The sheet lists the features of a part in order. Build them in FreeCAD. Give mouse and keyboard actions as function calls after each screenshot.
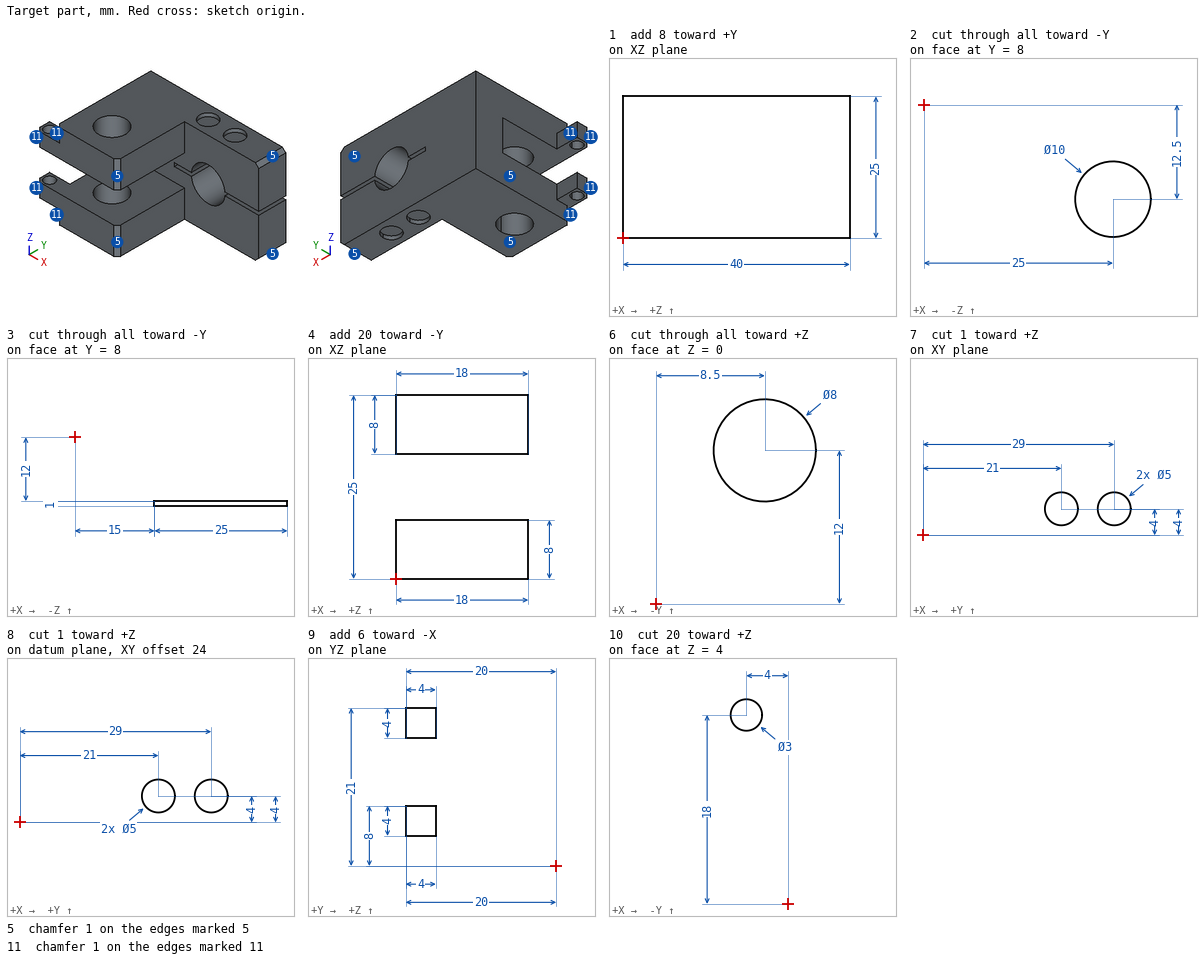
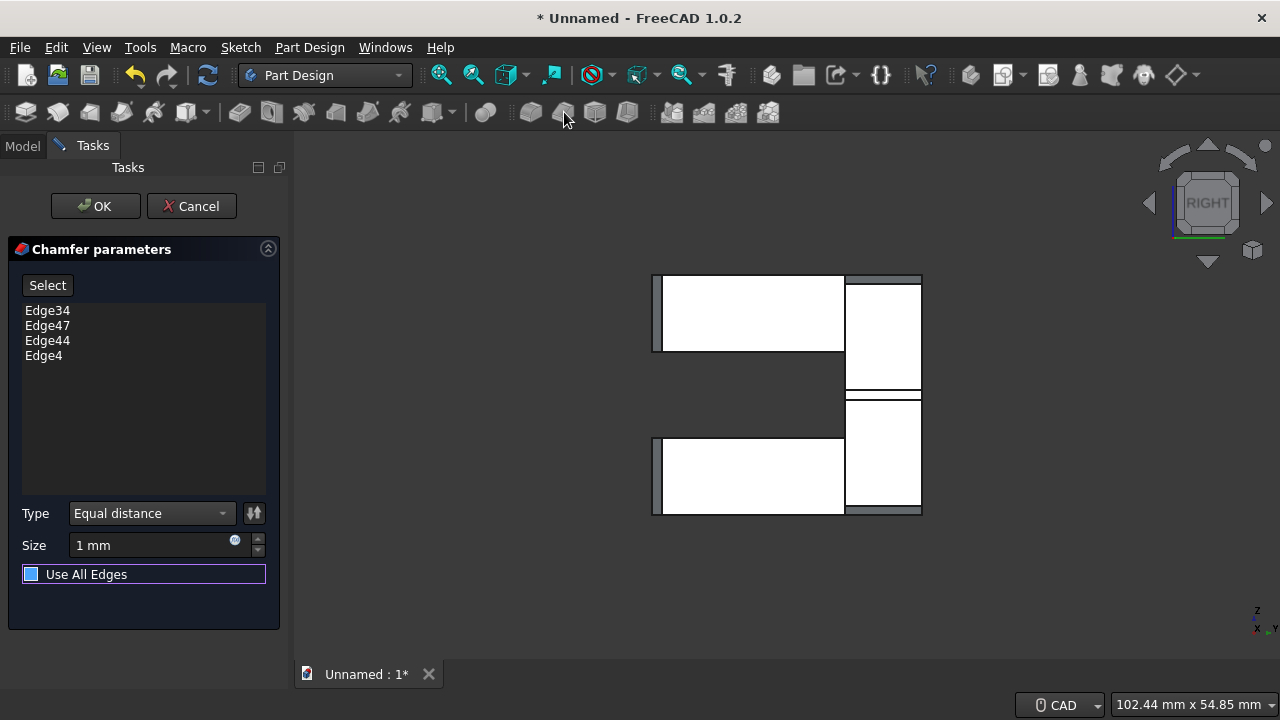
click(96, 206)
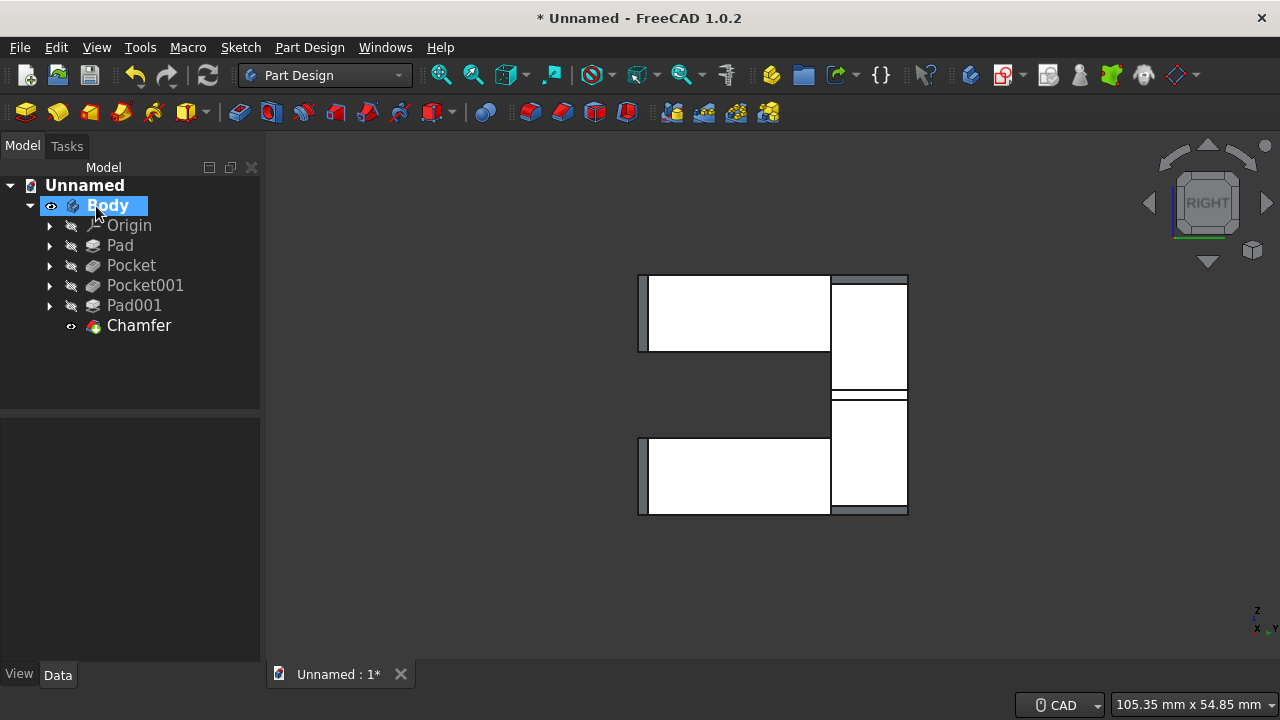
key(5)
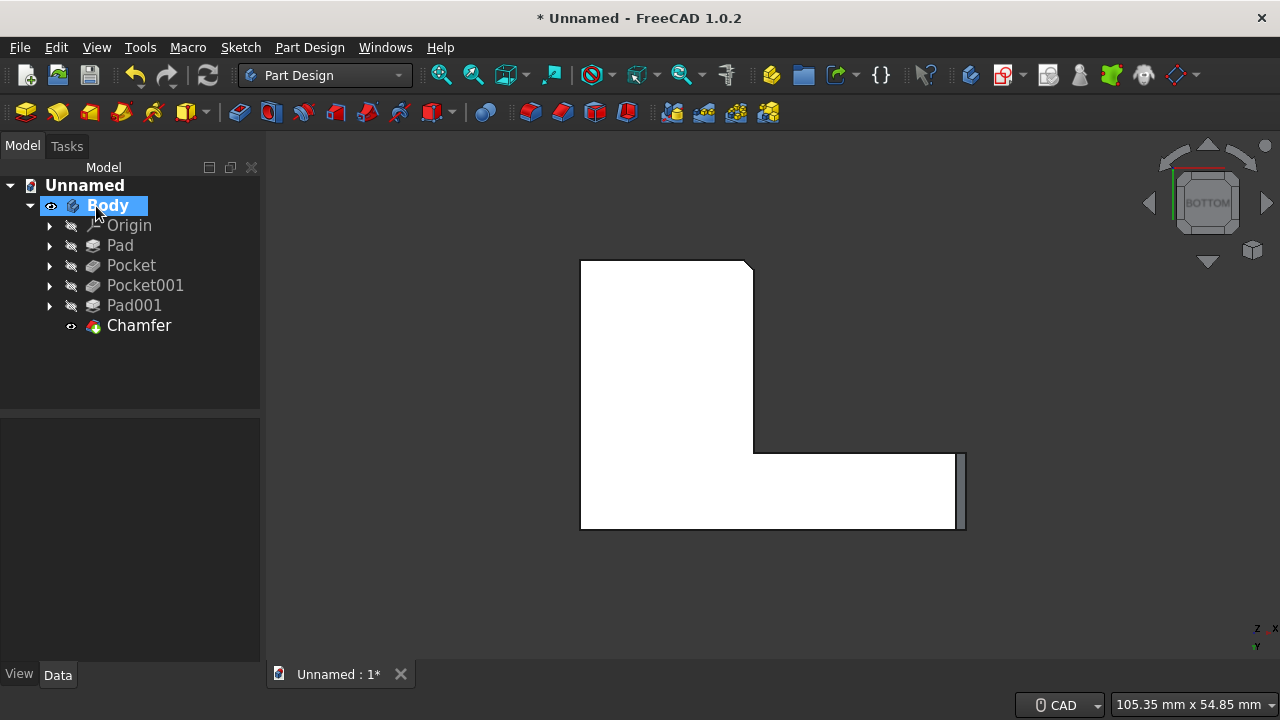
click(661, 433)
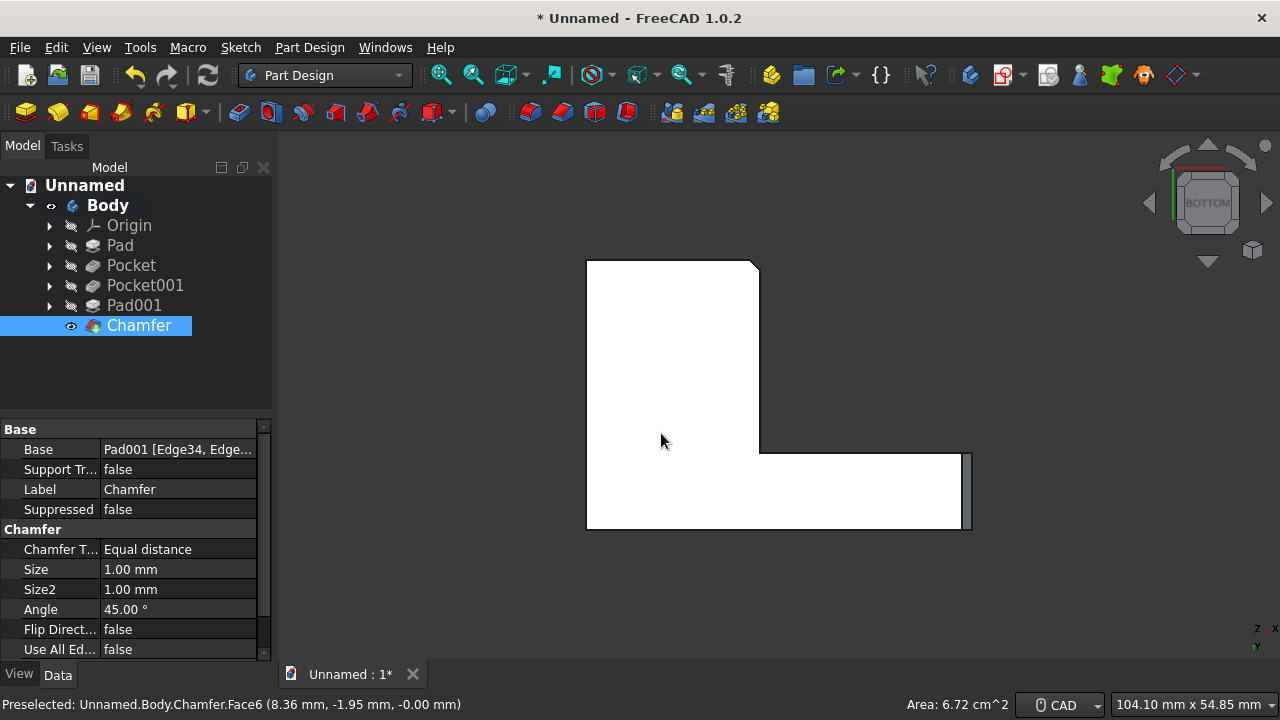
click(1004, 76)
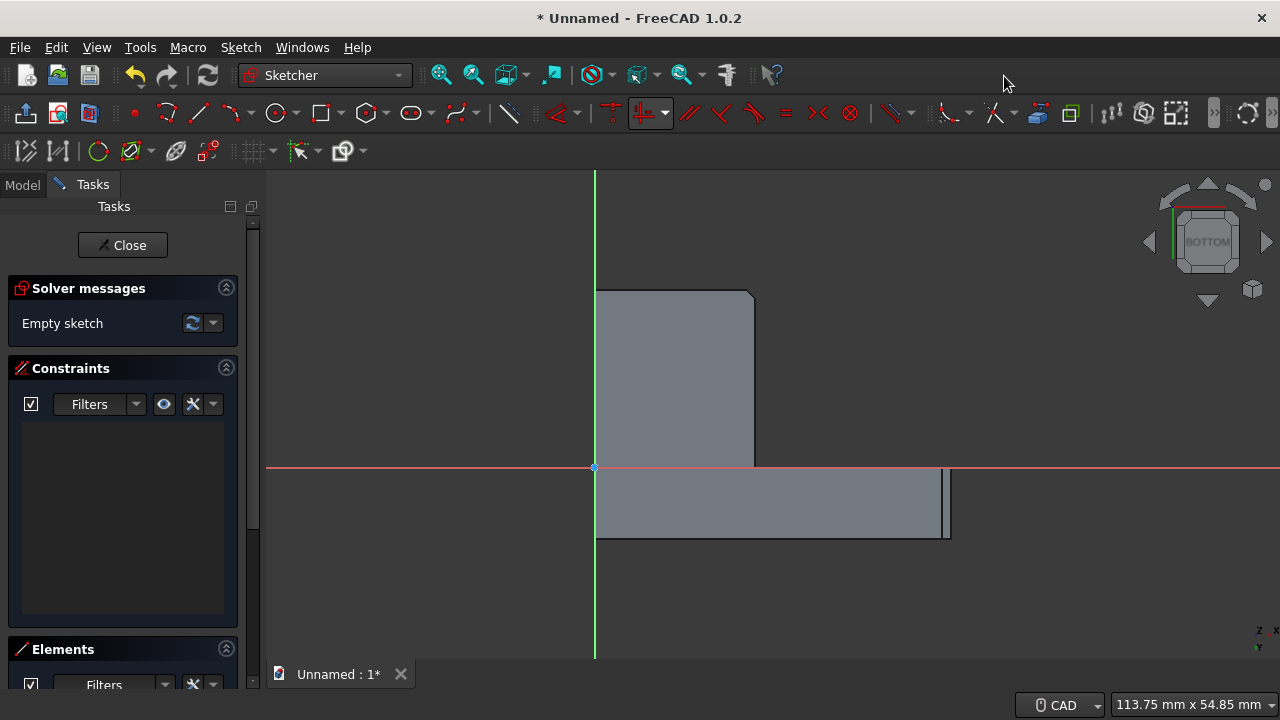
scroll(606, 382, up, 4)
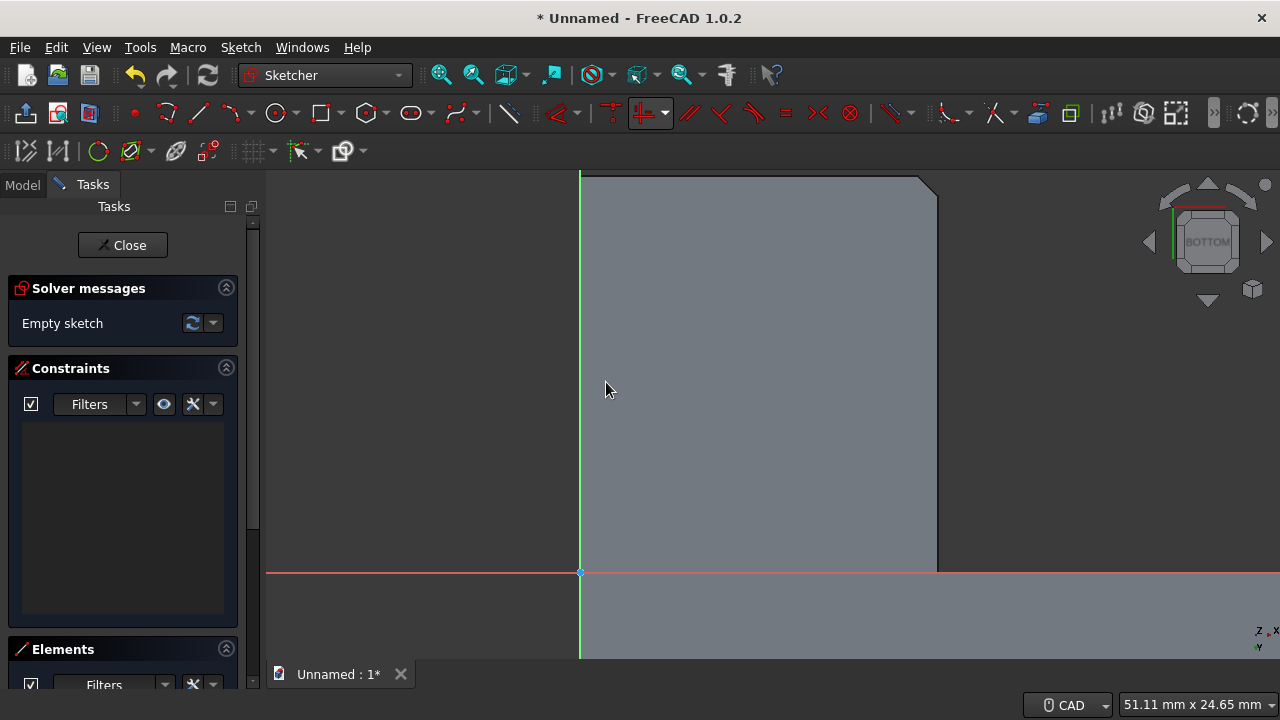
click(276, 114)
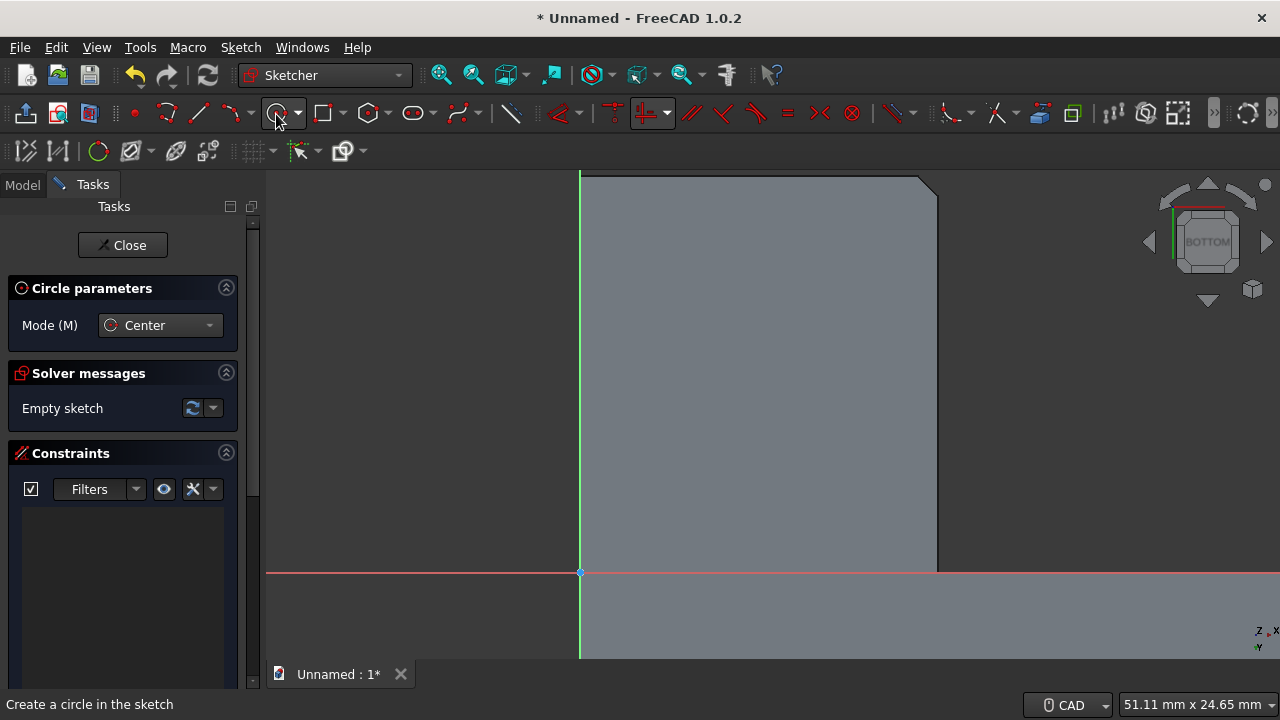
click(749, 335)
click(805, 279)
key(Escape)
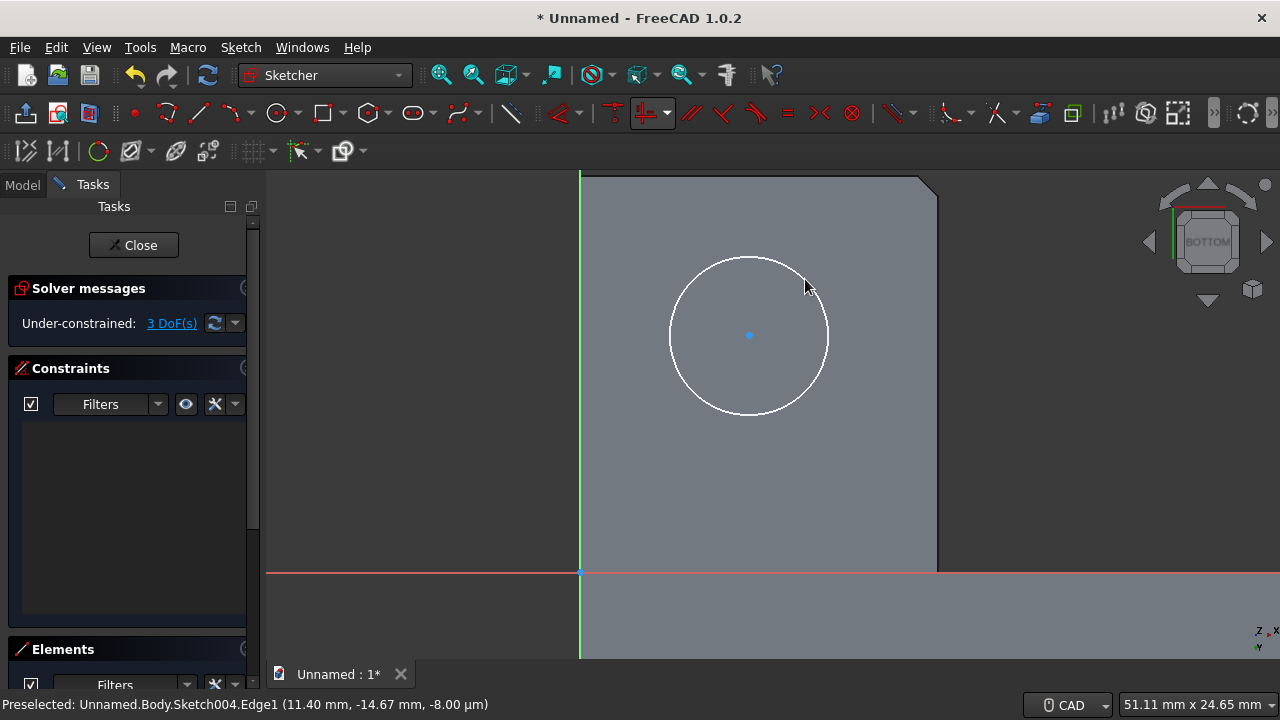
click(558, 114)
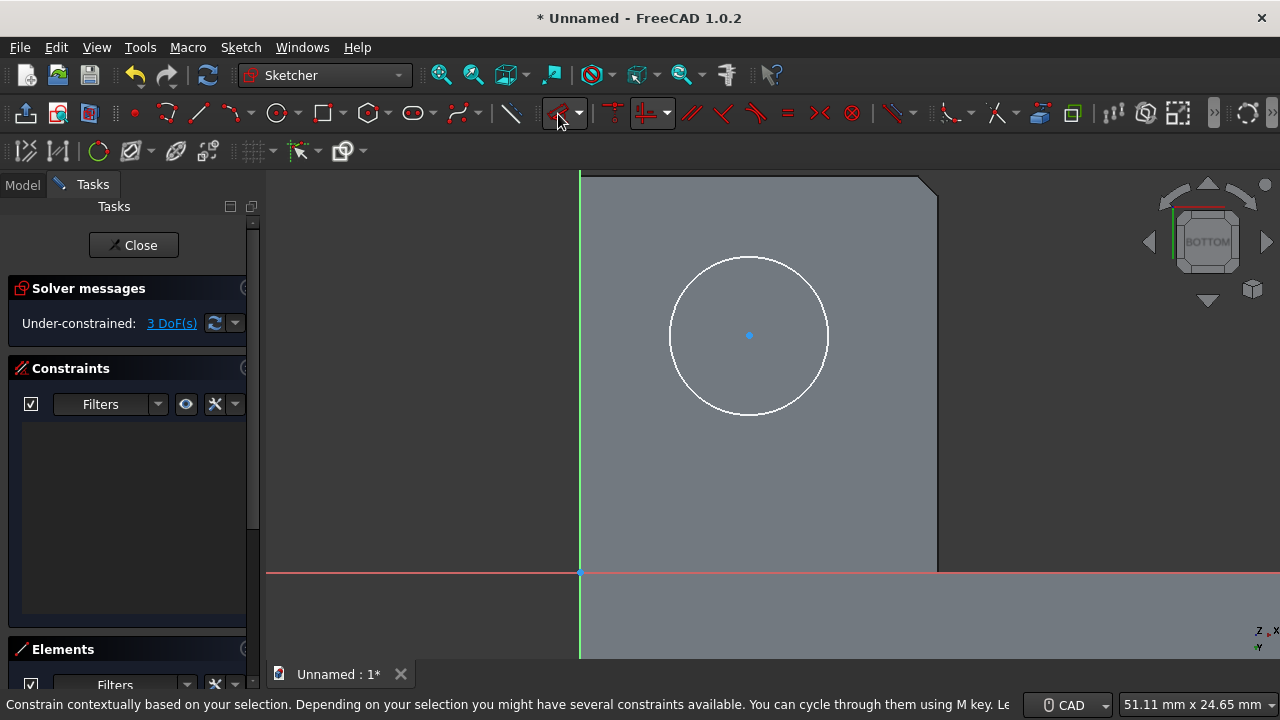
click(805, 280)
click(828, 257)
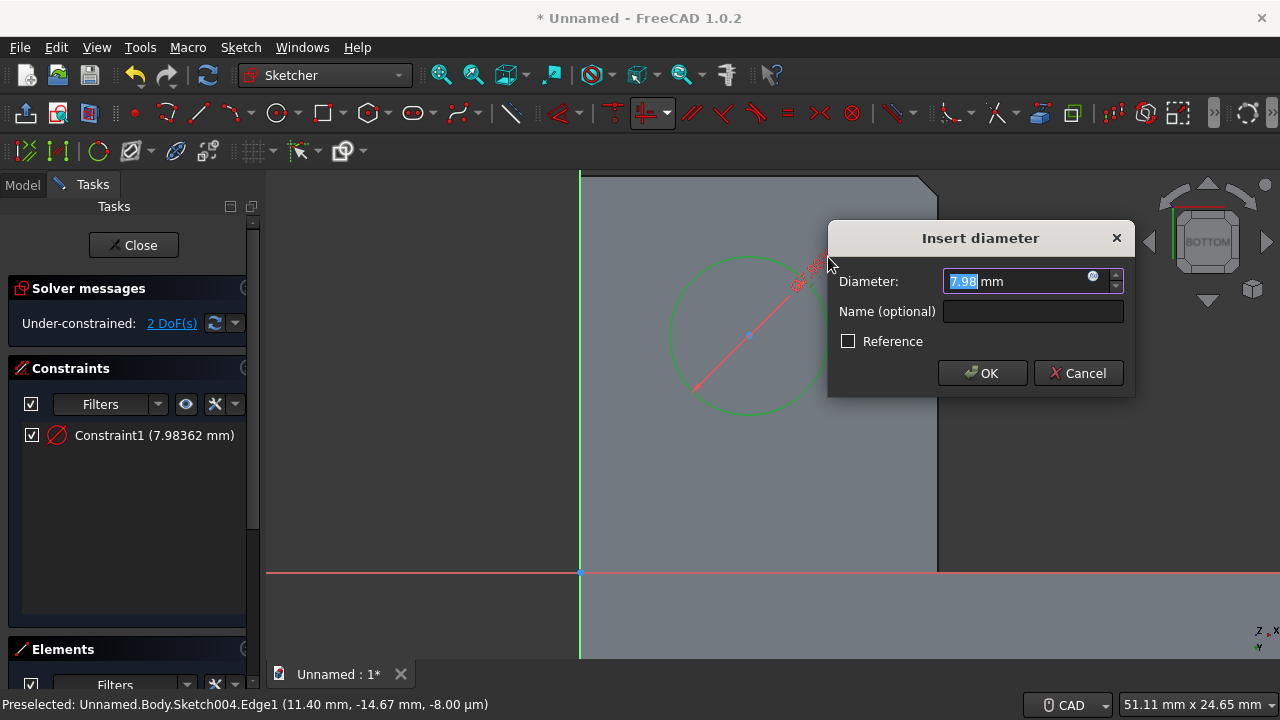
text(8)
key(Return)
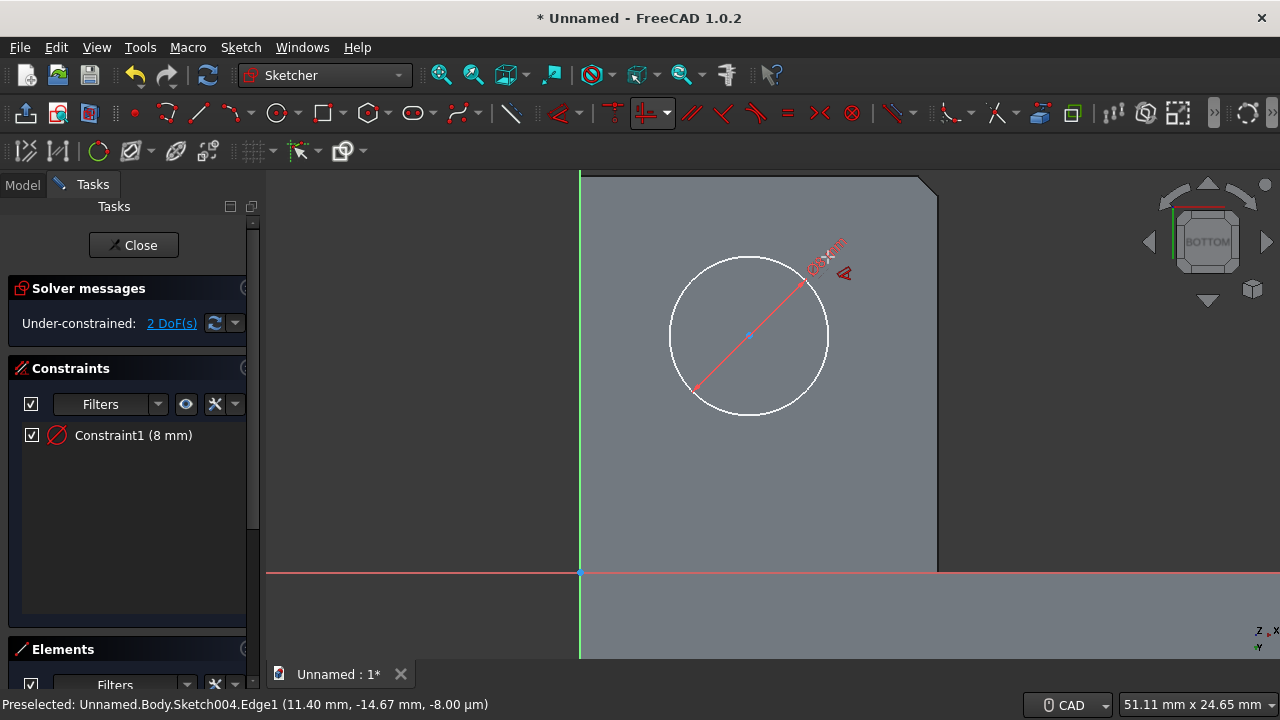
click(749, 336)
click(546, 454)